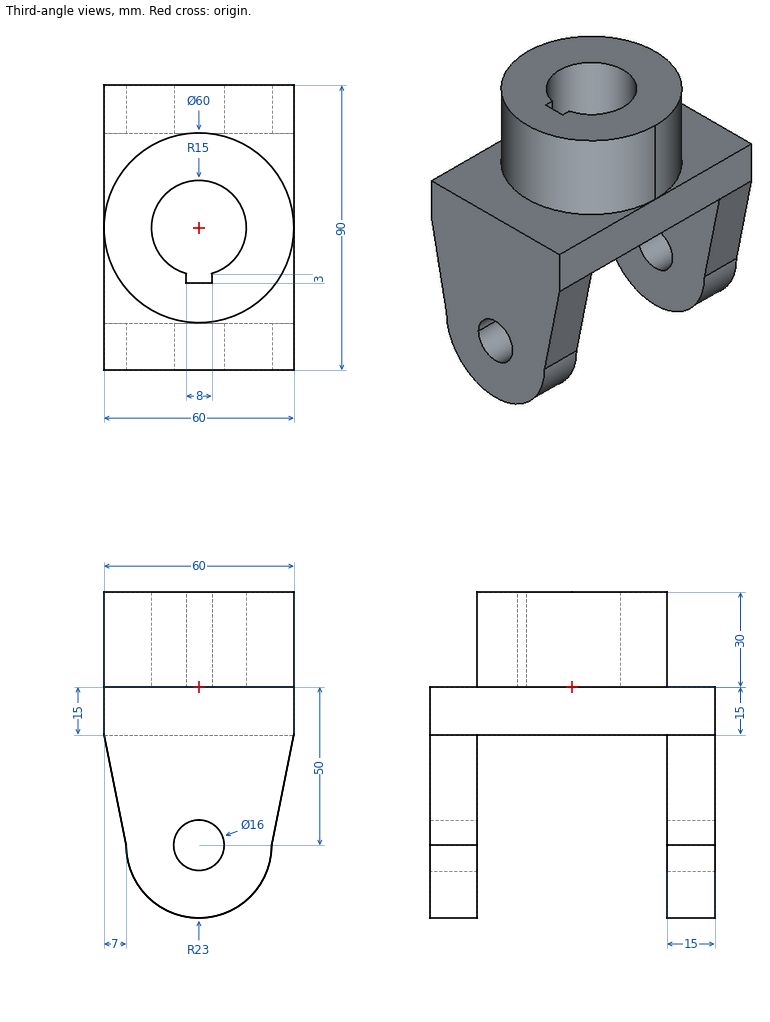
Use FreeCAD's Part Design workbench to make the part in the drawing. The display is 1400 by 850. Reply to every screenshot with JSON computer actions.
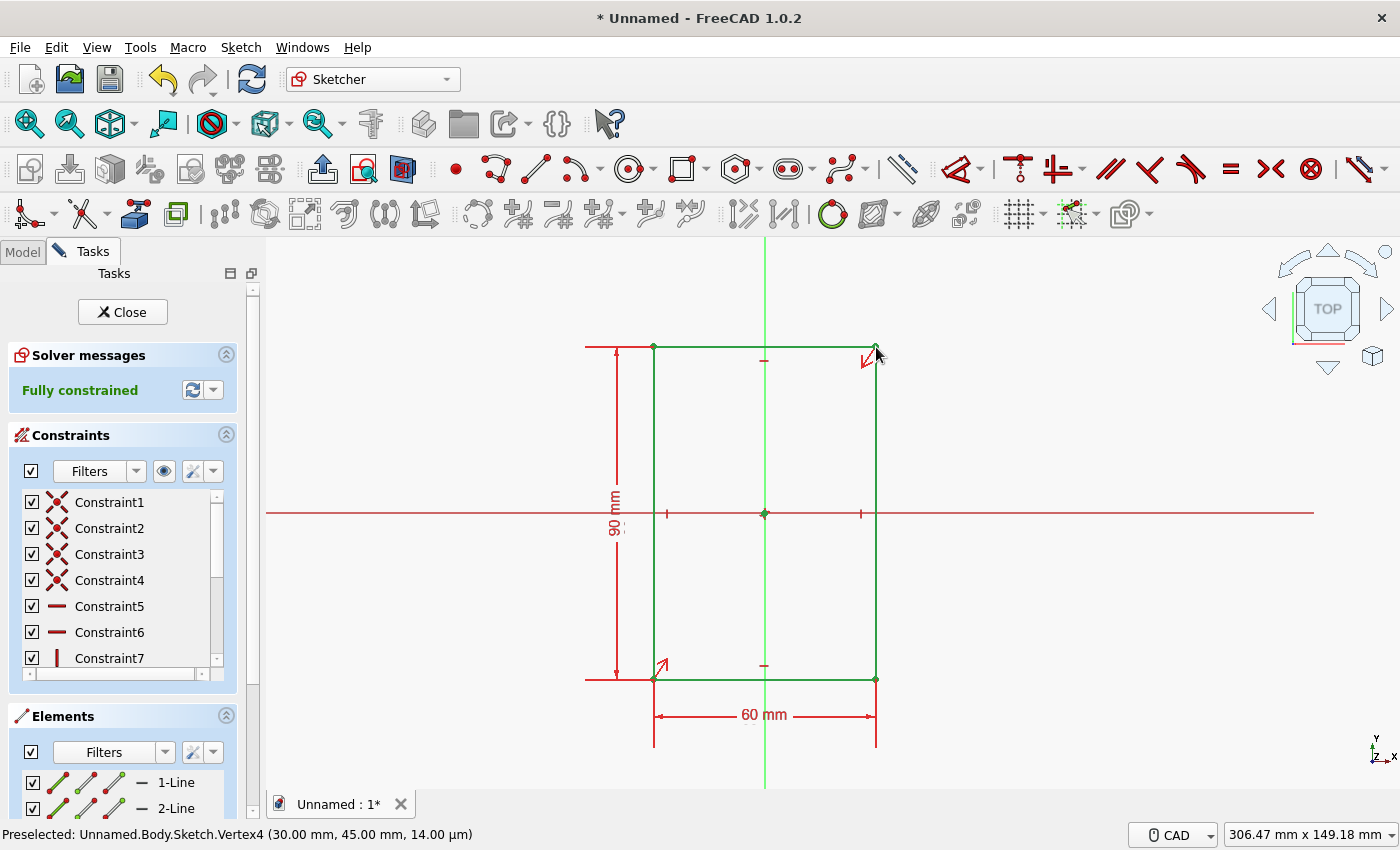
{"action": "left_click", "coordinate": [123, 312]}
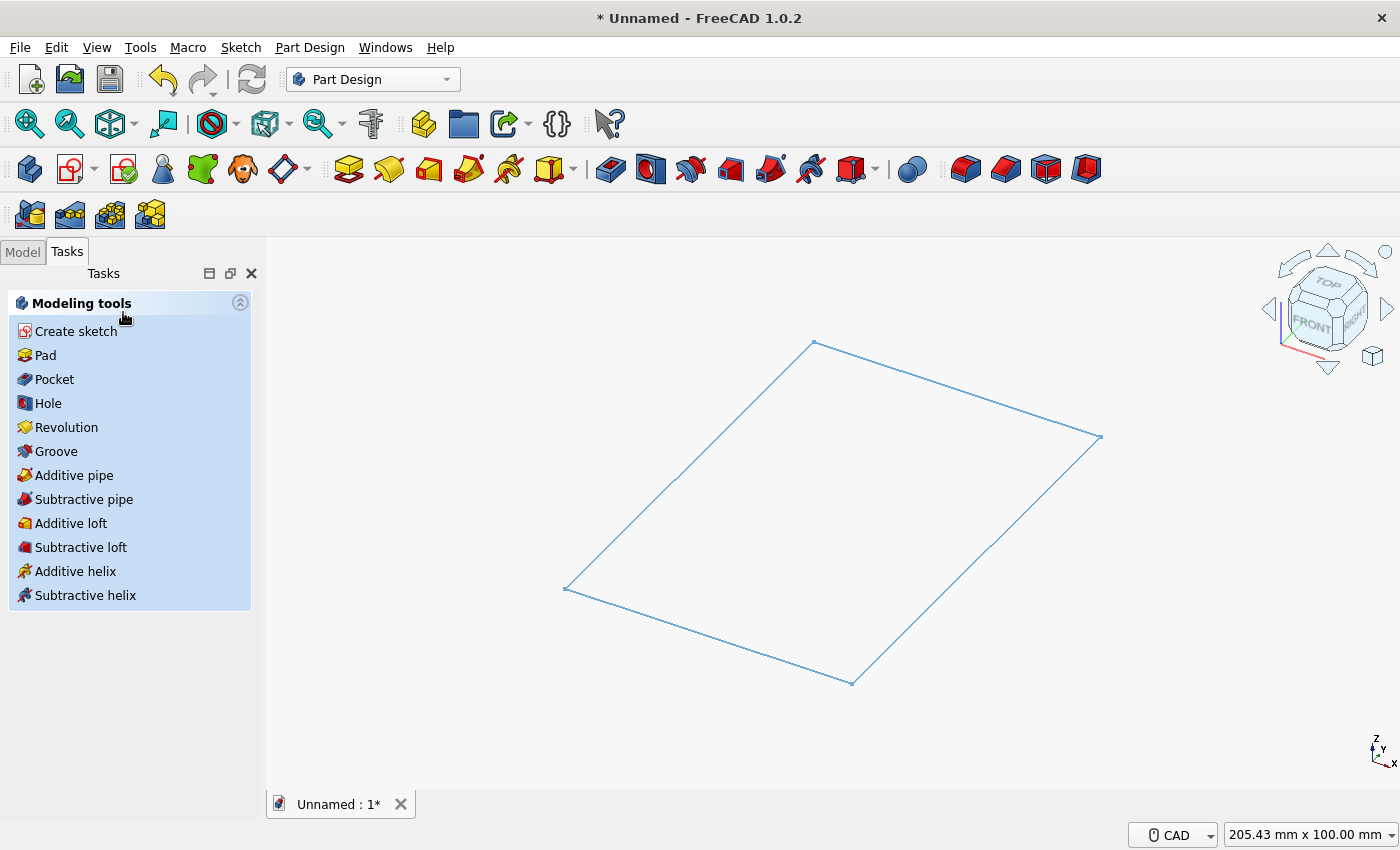
{"action": "left_click", "coordinate": [350, 170]}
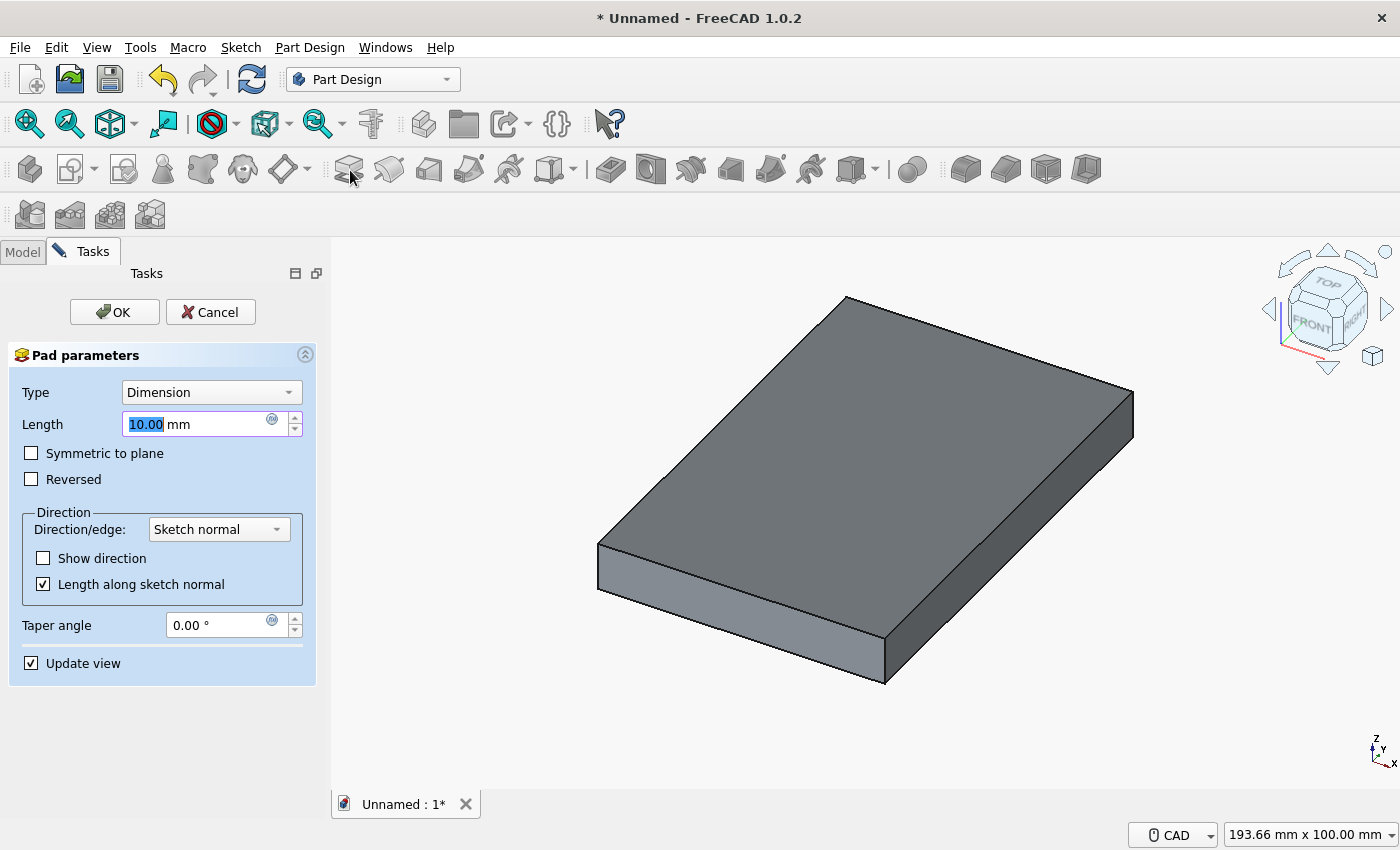
{"action": "type", "text": "15"}
{"action": "key", "text": "Tab"}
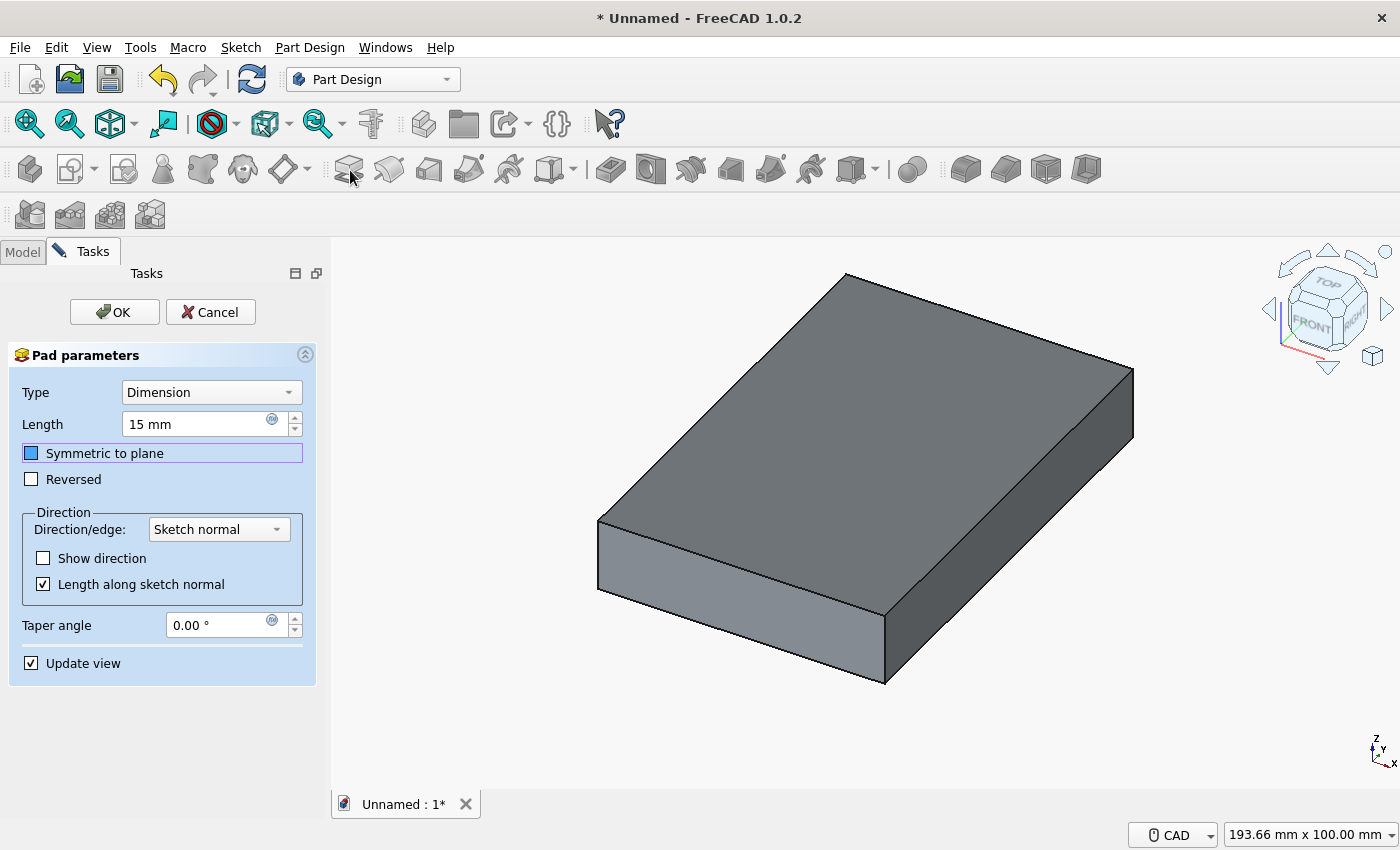
{"action": "left_click", "coordinate": [30, 479]}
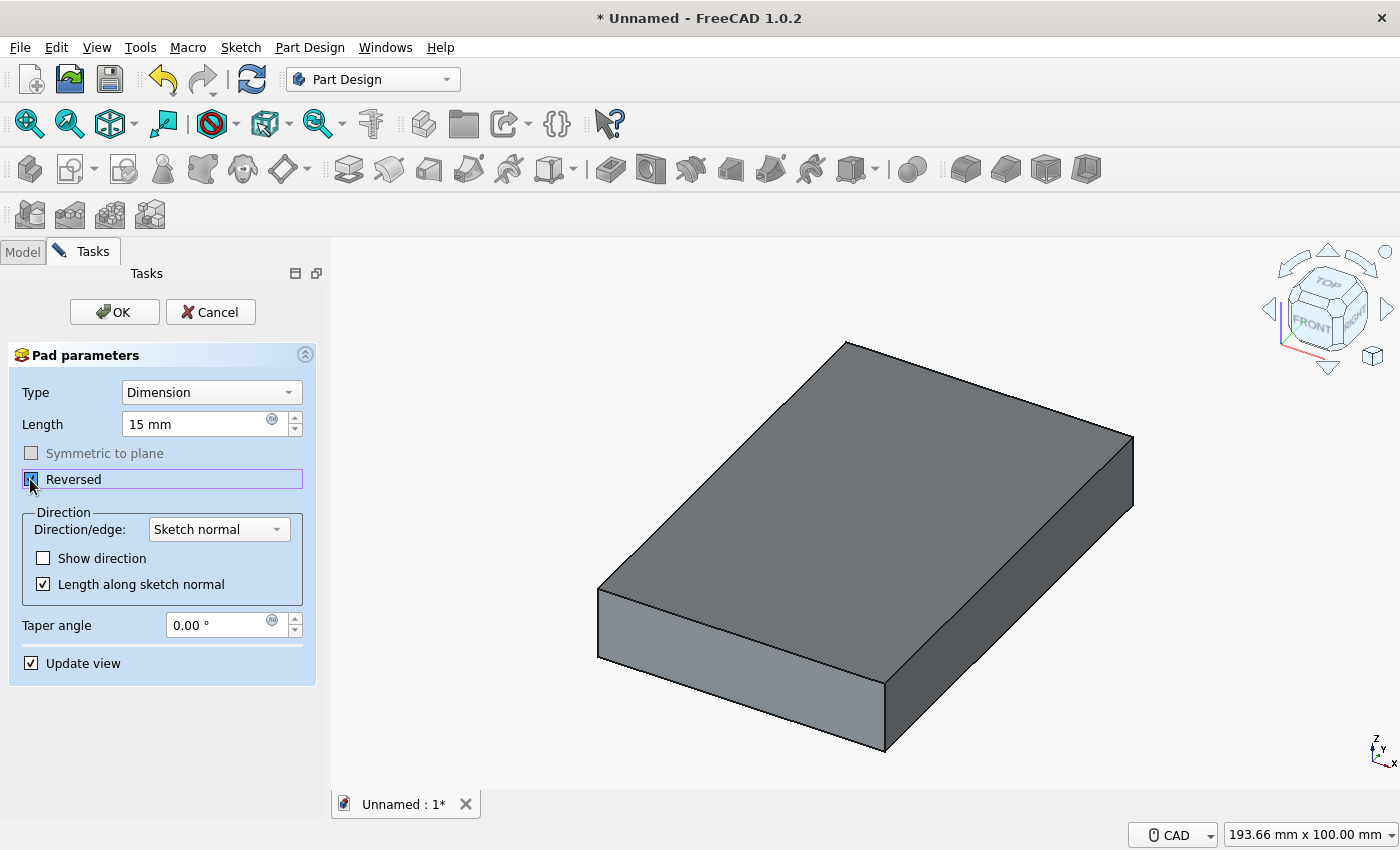
{"action": "left_click", "coordinate": [115, 312]}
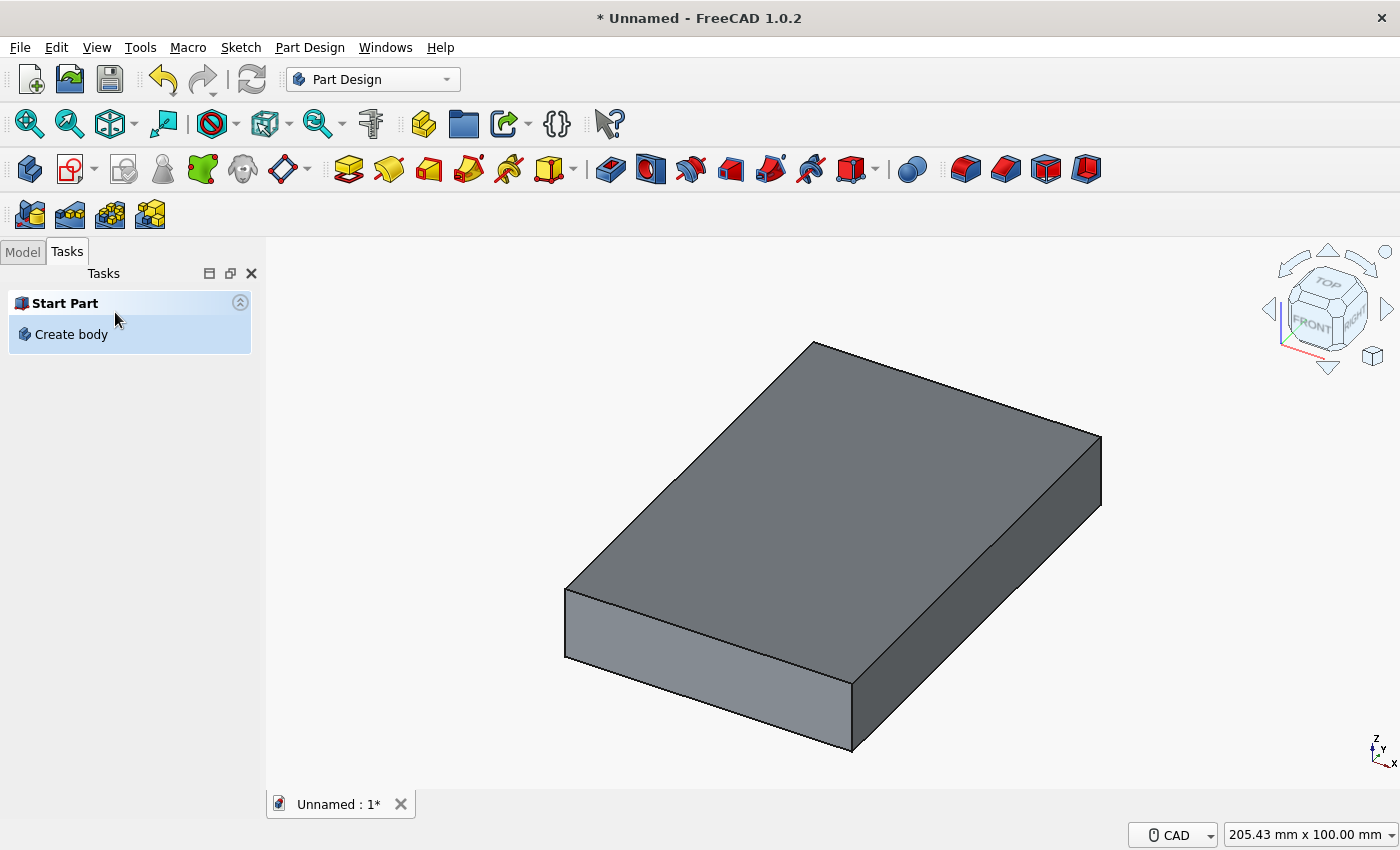
{"action": "key", "text": "4"}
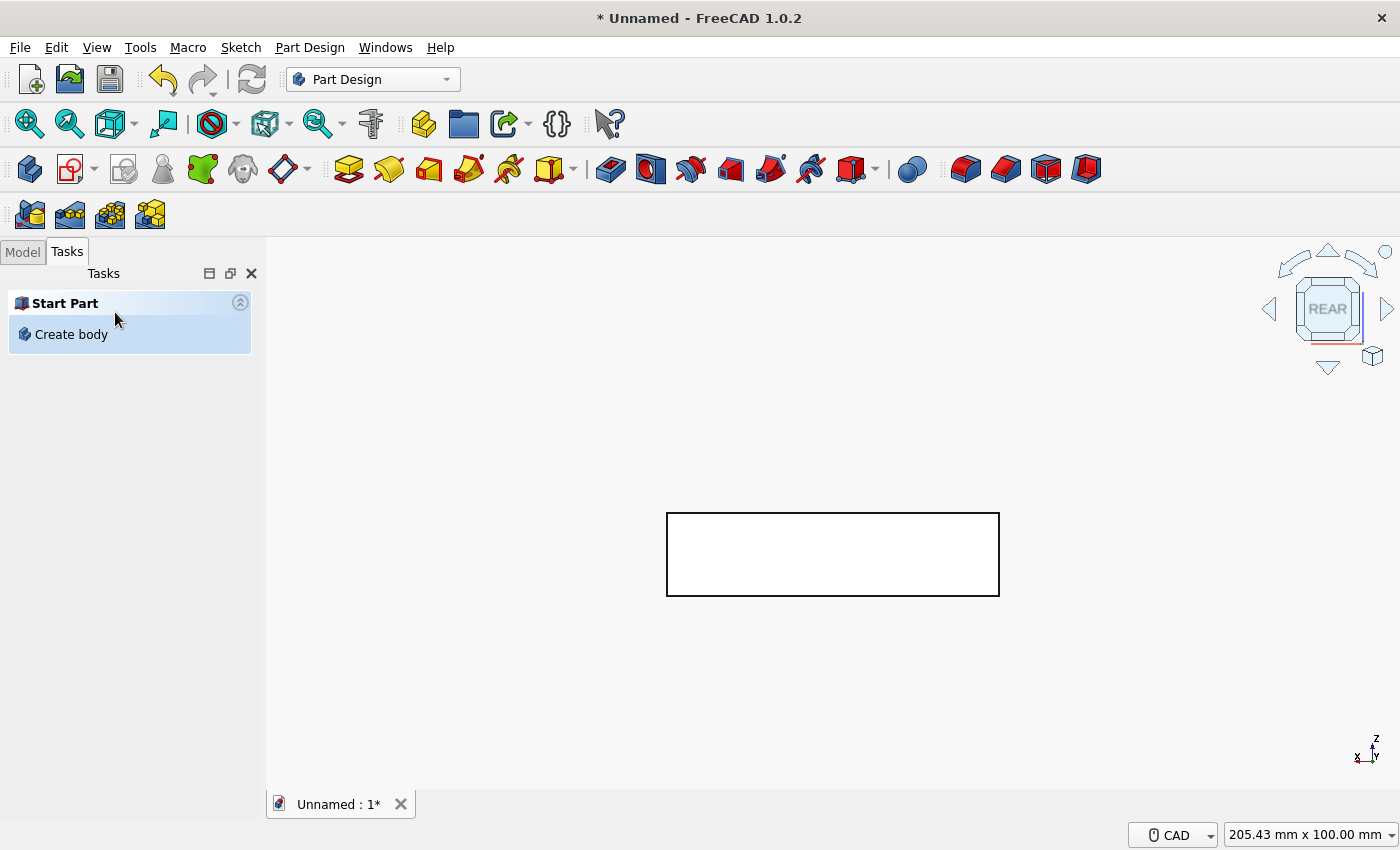
{"action": "left_click", "coordinate": [30, 124]}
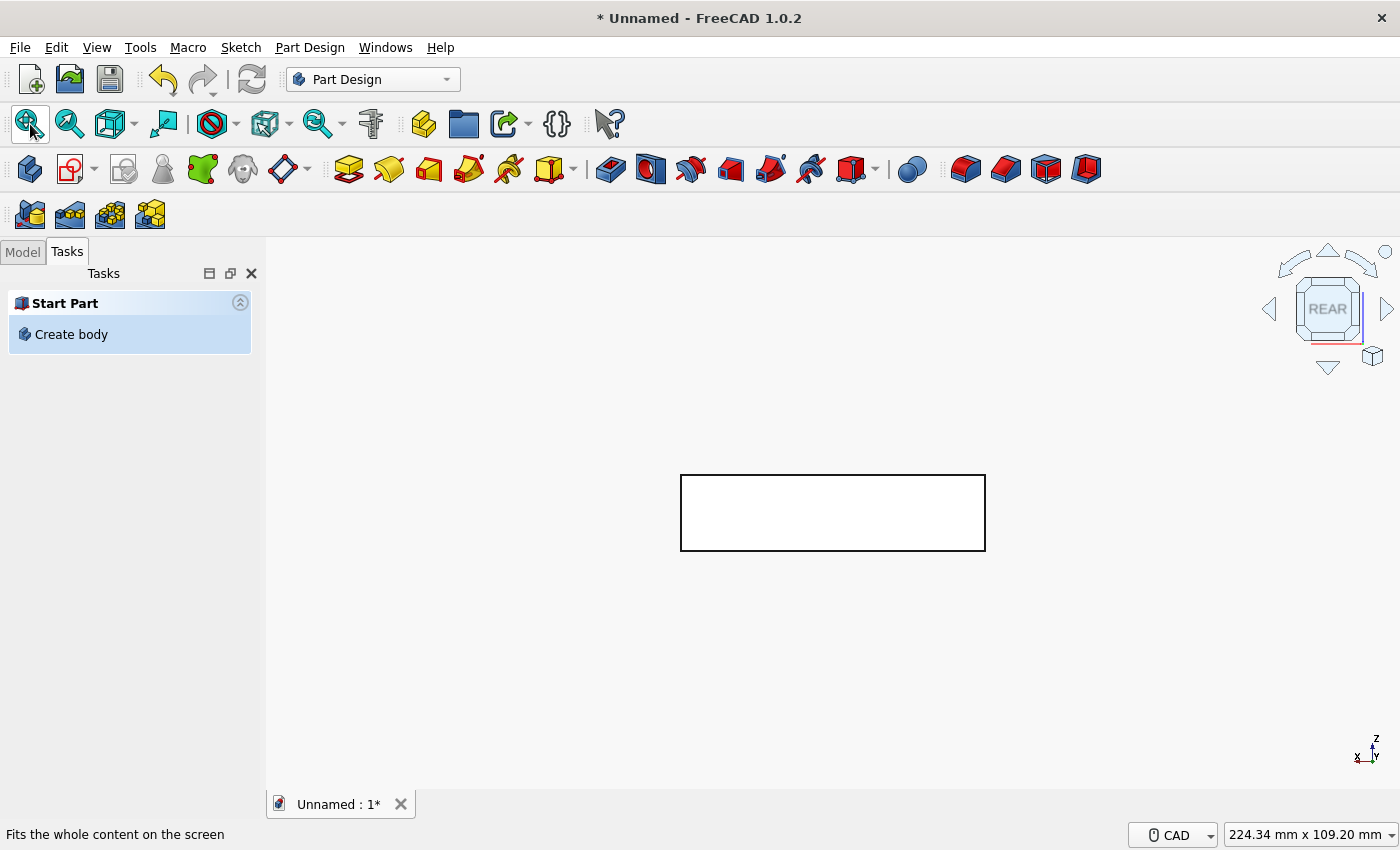
{"action": "left_click", "coordinate": [746, 512]}